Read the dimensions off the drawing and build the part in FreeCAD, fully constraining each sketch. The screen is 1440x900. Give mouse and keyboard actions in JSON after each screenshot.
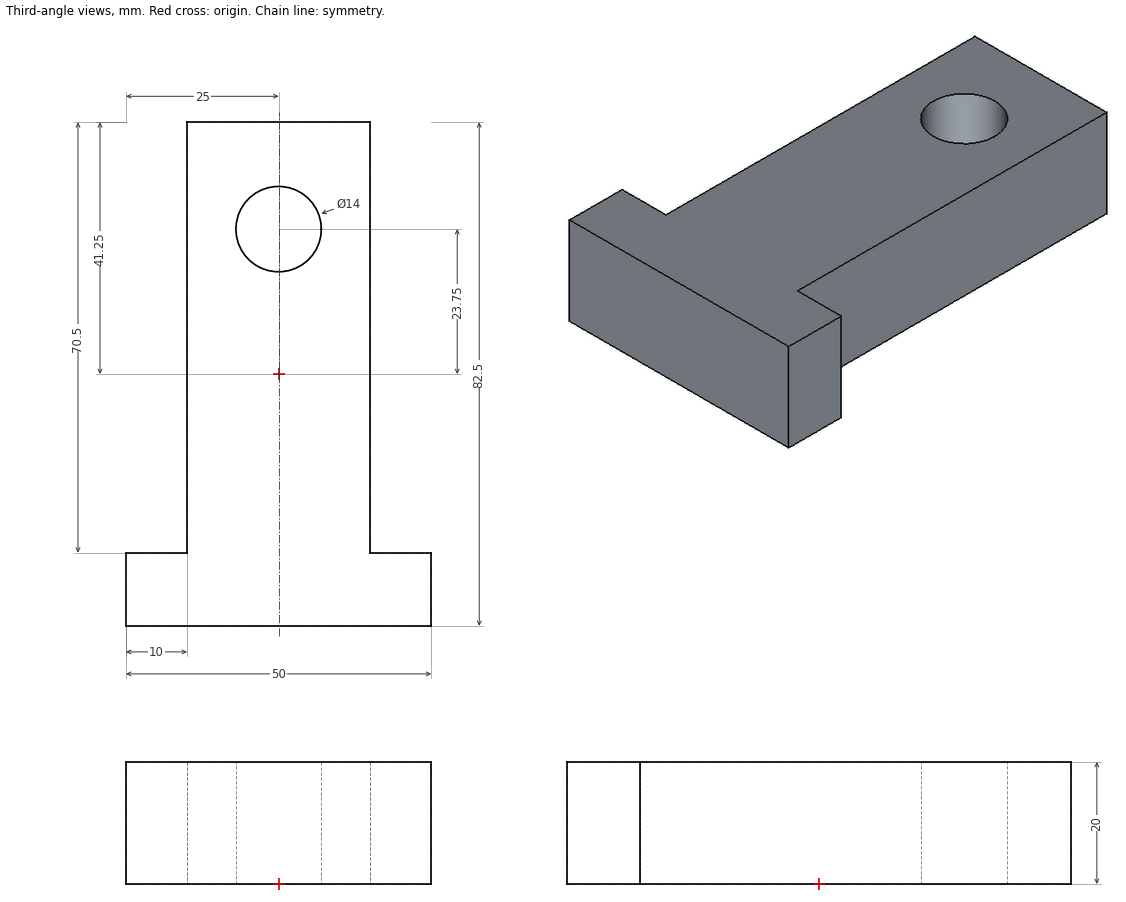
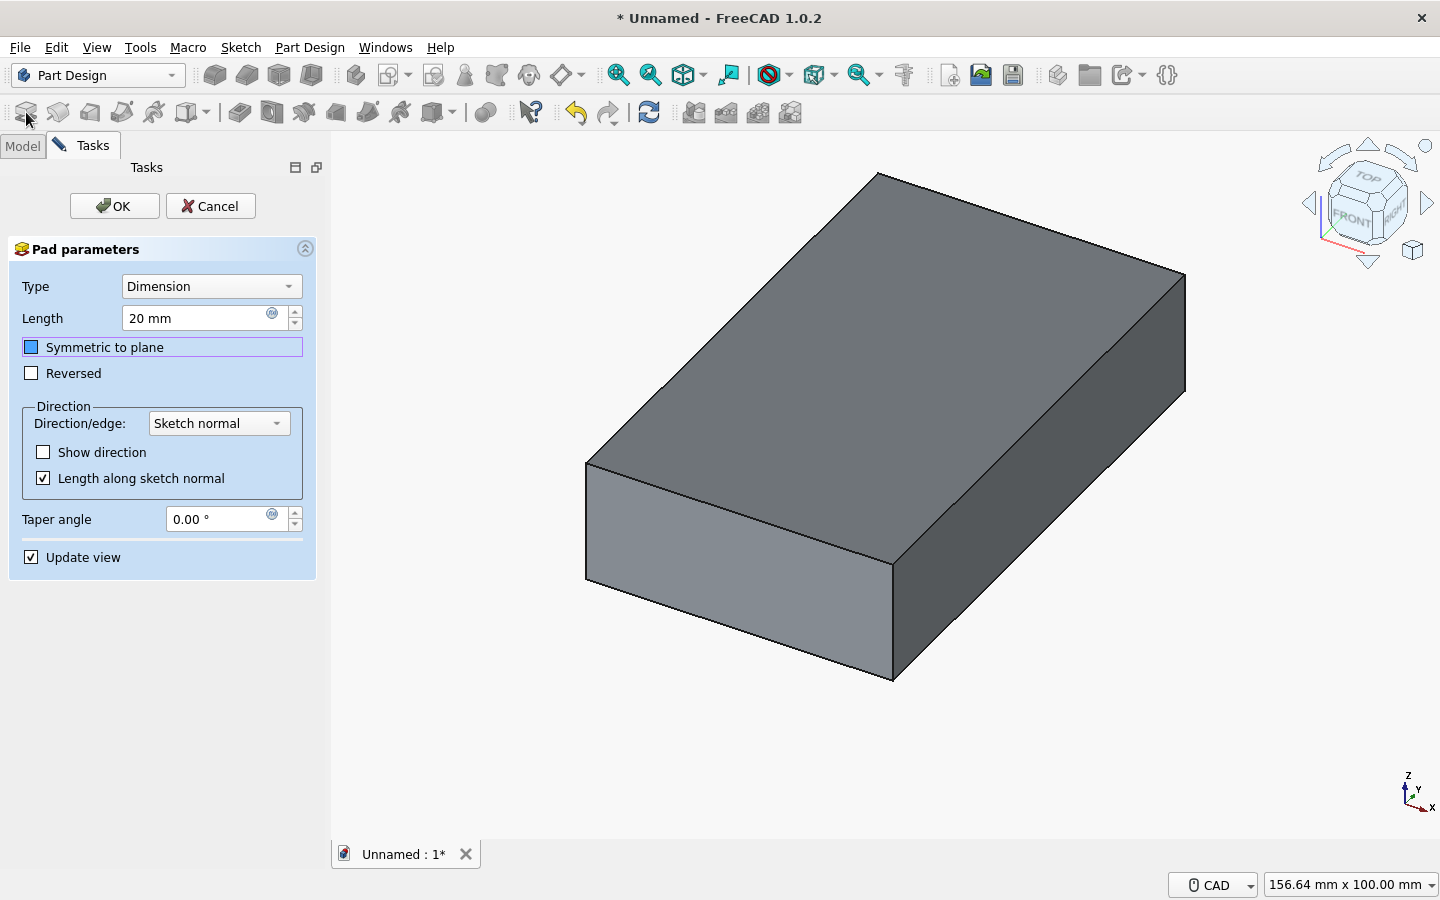
{"action": "left_click", "coordinate": [115, 206]}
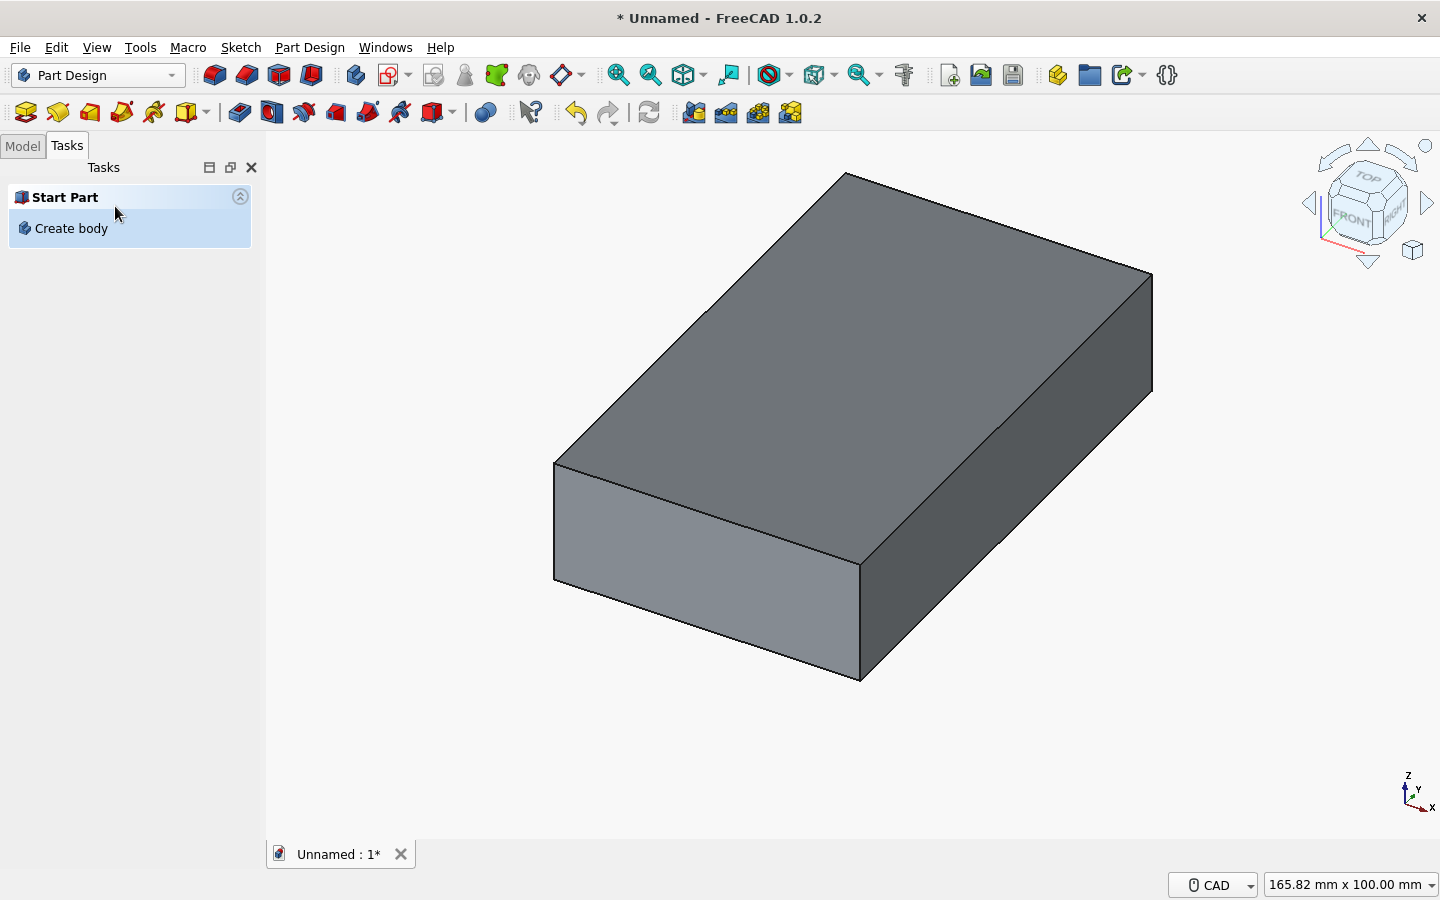
{"action": "left_click", "coordinate": [895, 327]}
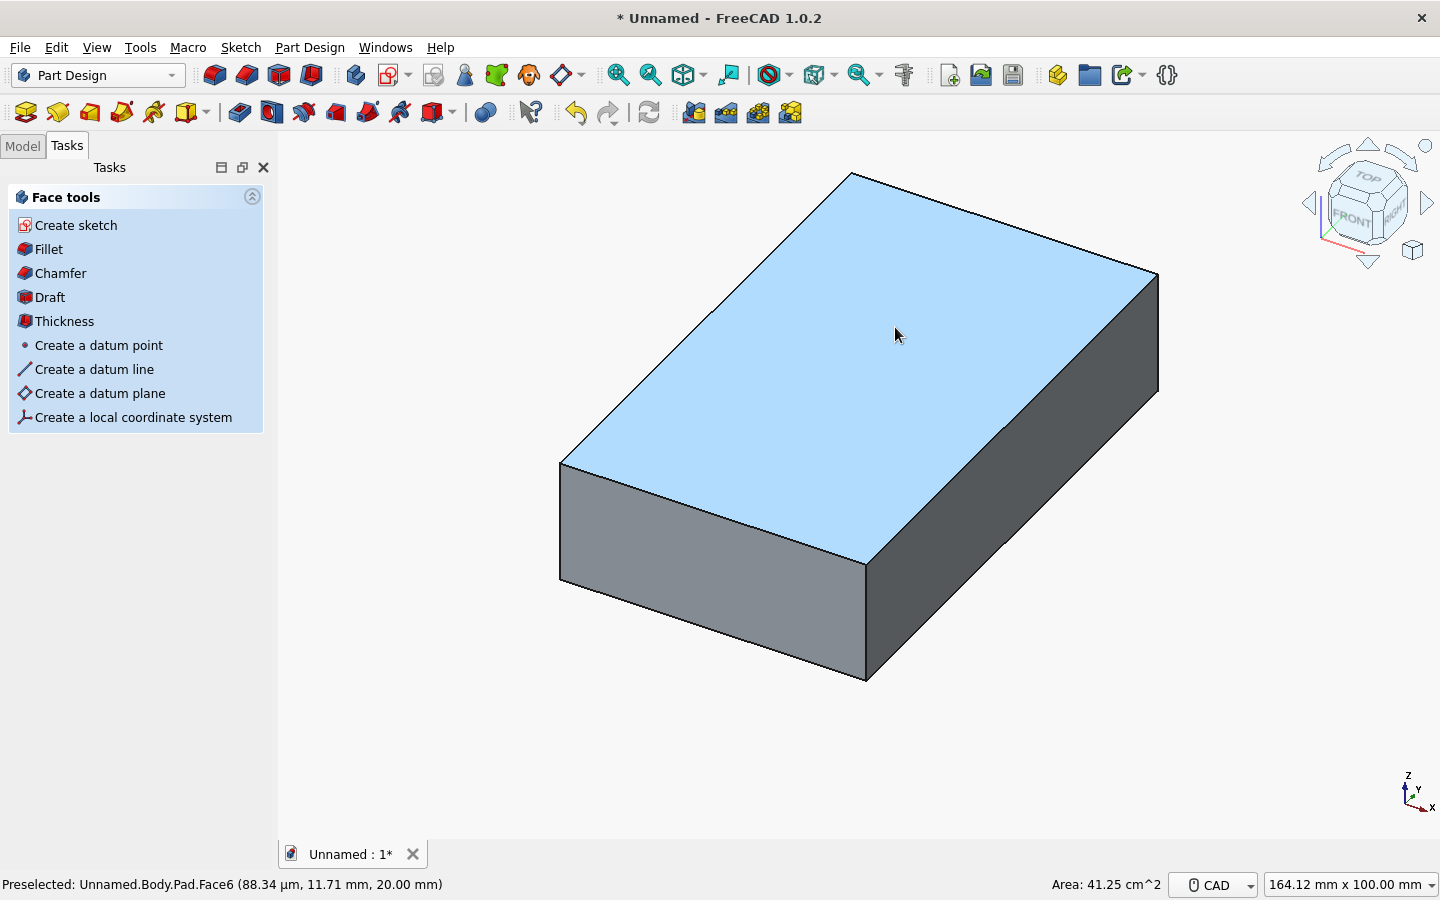
{"action": "left_click", "coordinate": [388, 76]}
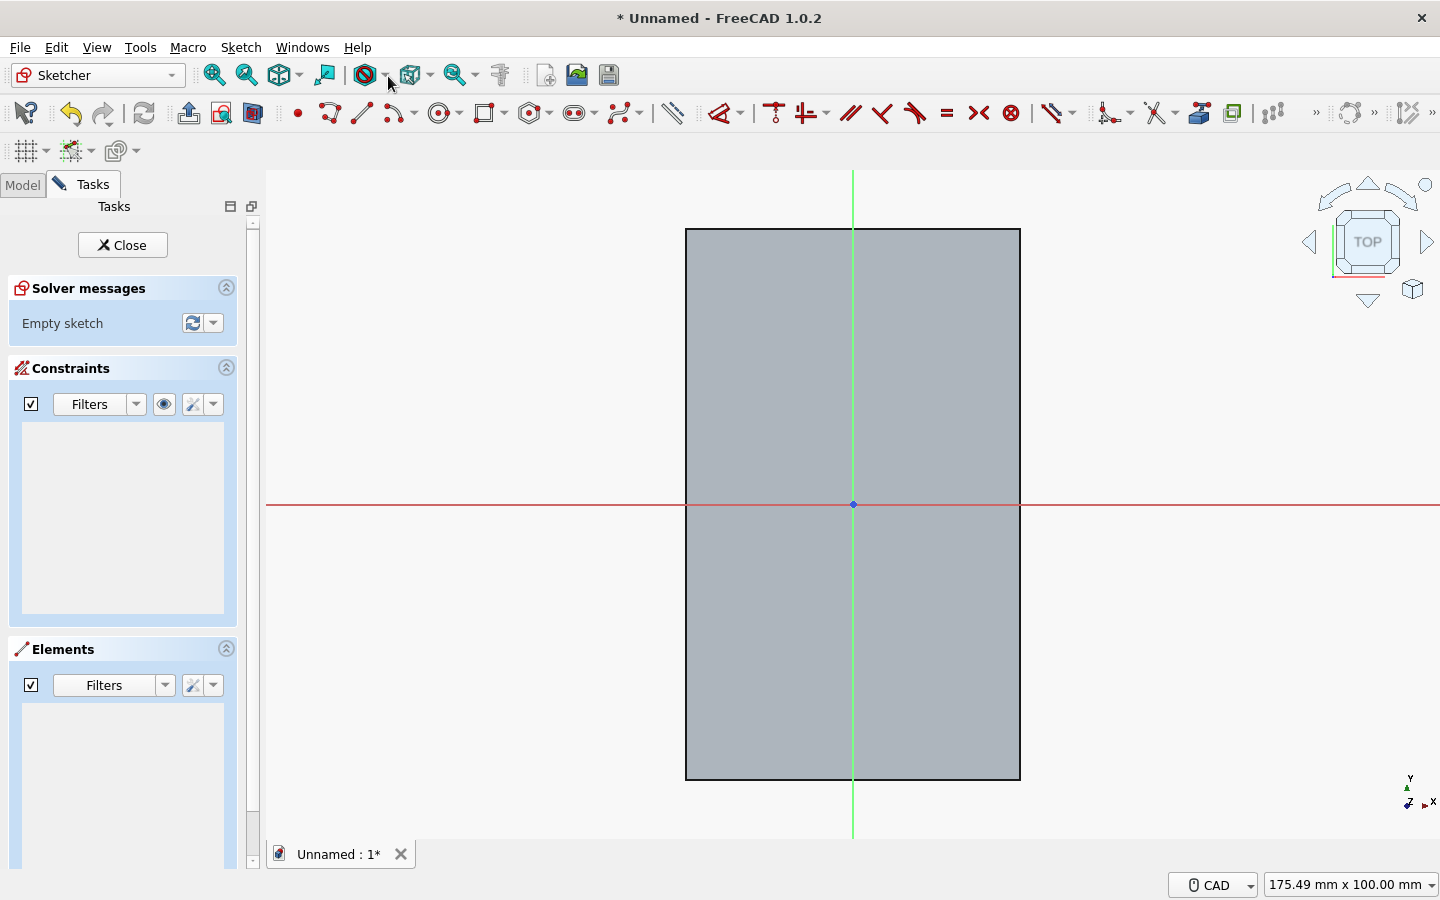
{"action": "scroll", "coordinate": [909, 318], "scroll_direction": "up", "scroll_amount": 4}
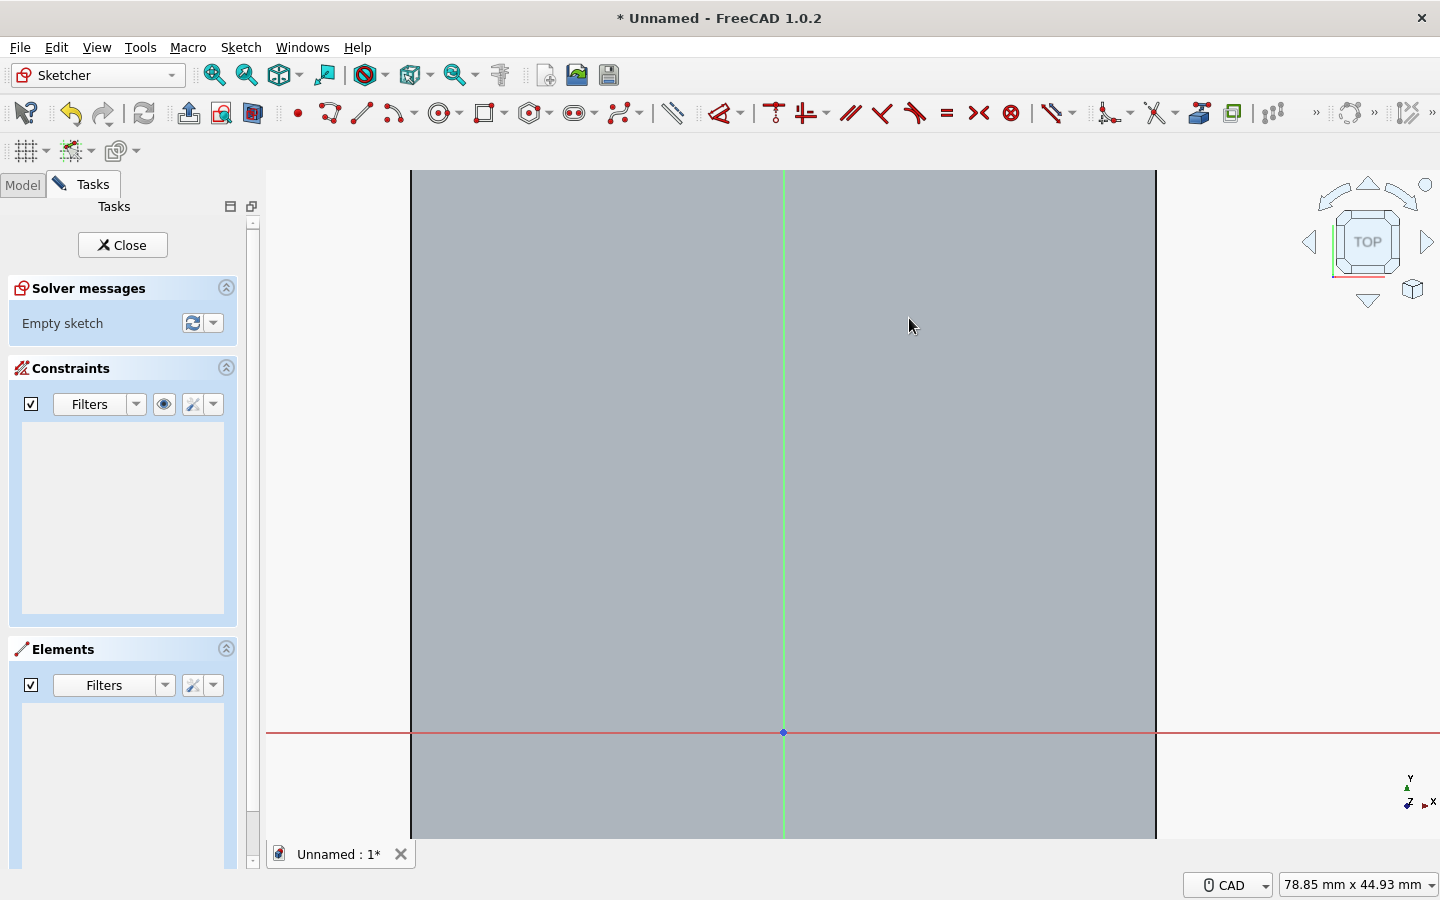
{"action": "left_click", "coordinate": [440, 114]}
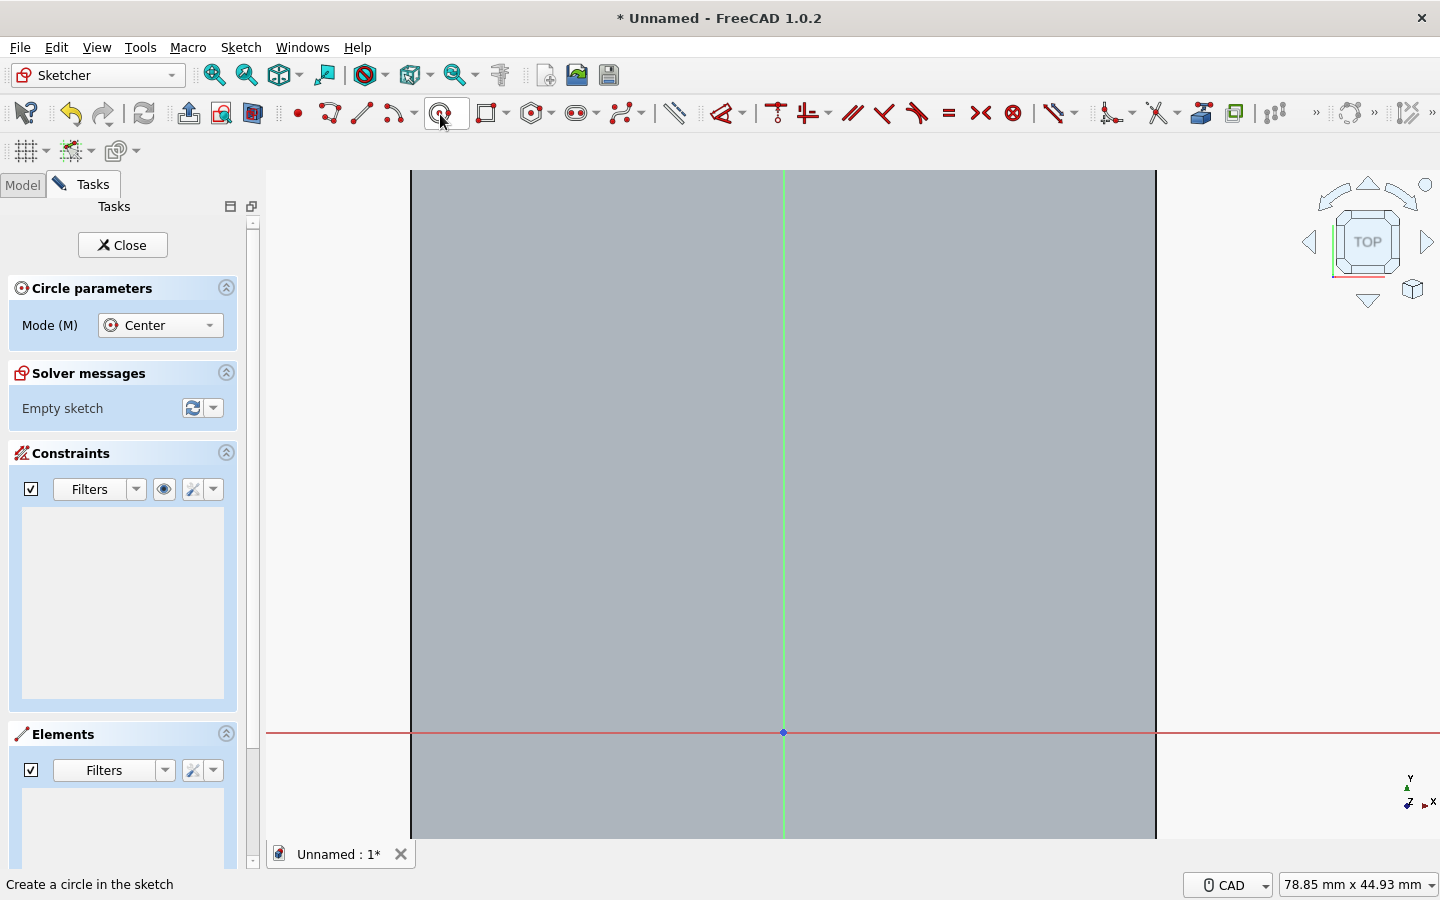
{"action": "left_click", "coordinate": [784, 379]}
{"action": "left_click", "coordinate": [857, 305]}
{"action": "key", "text": "Escape"}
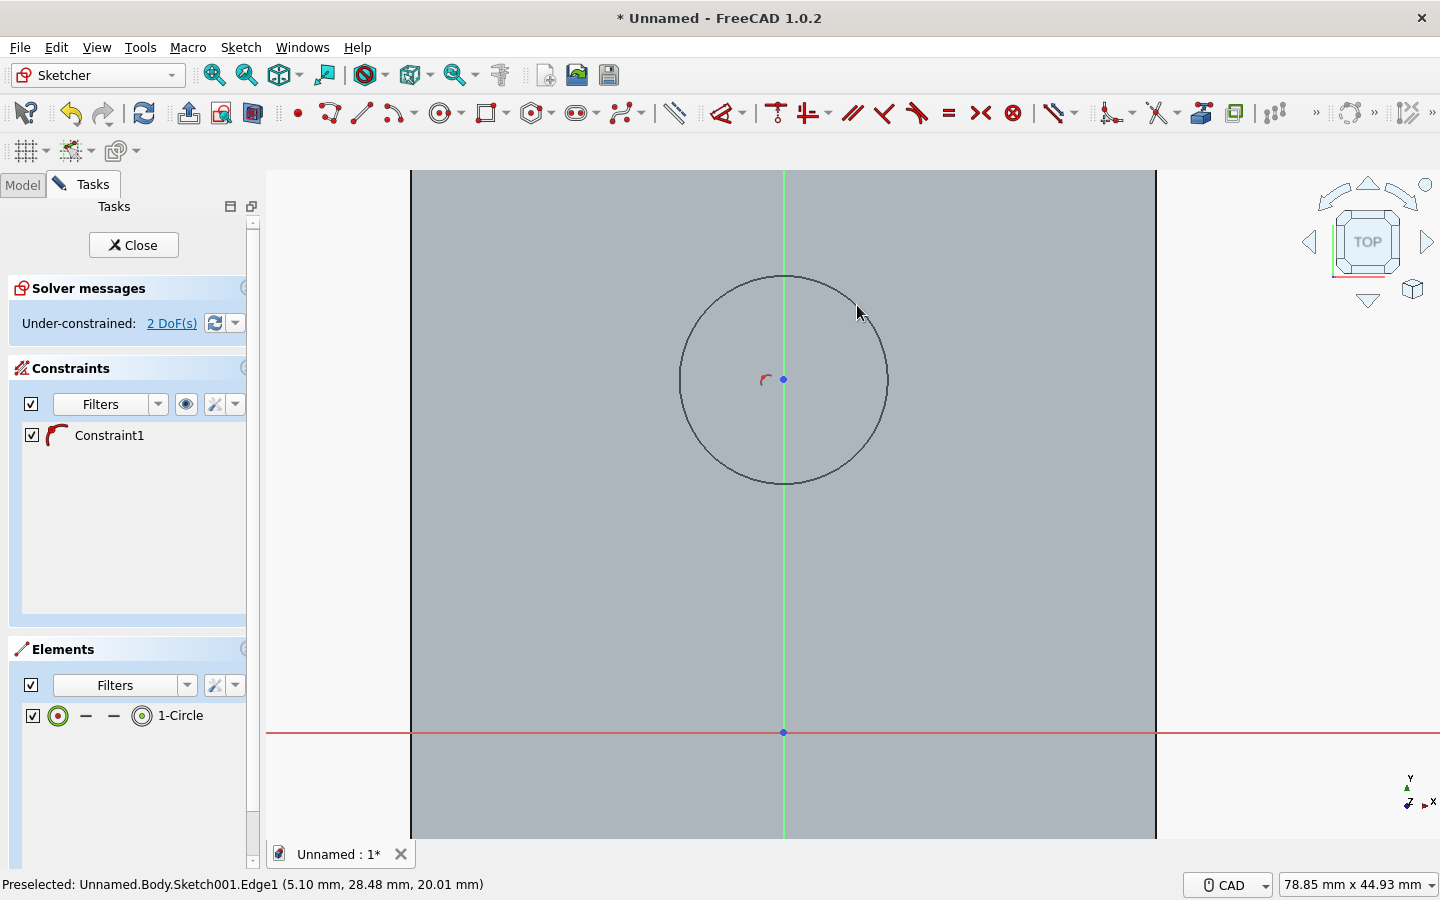
{"action": "left_click", "coordinate": [722, 114]}